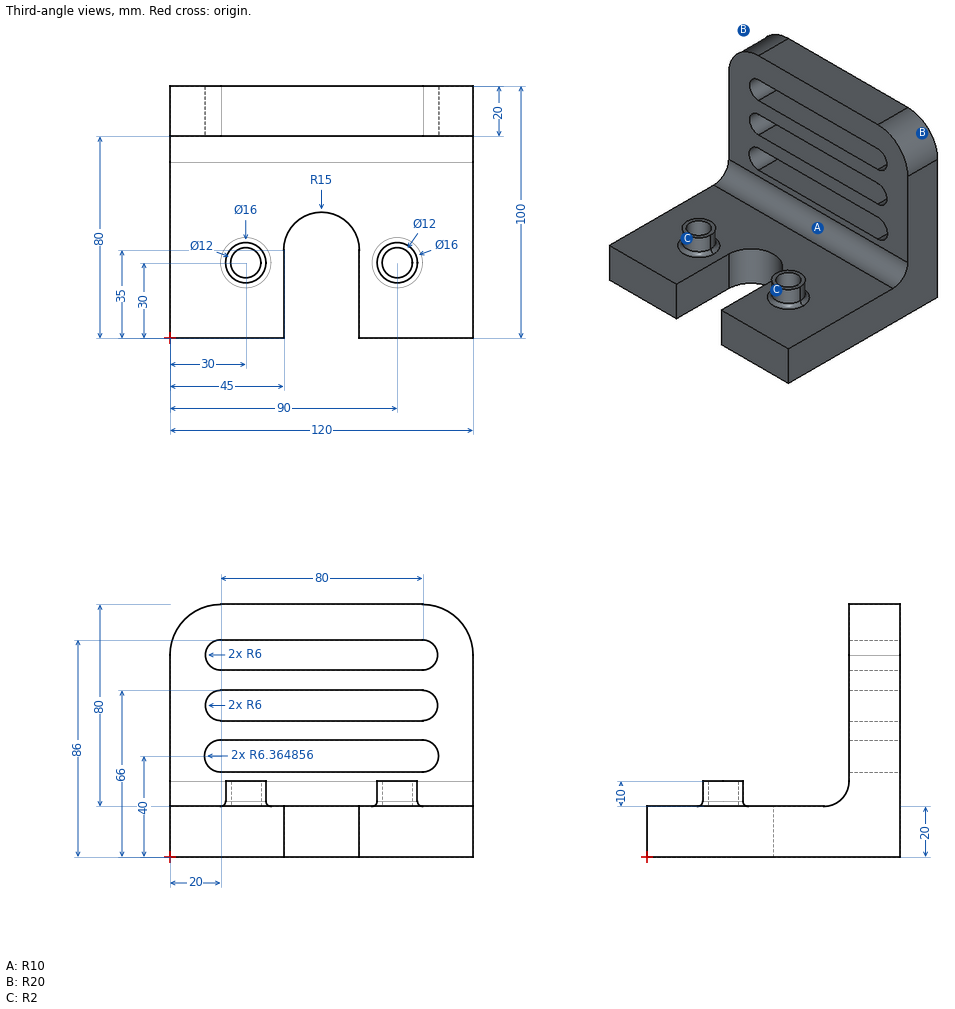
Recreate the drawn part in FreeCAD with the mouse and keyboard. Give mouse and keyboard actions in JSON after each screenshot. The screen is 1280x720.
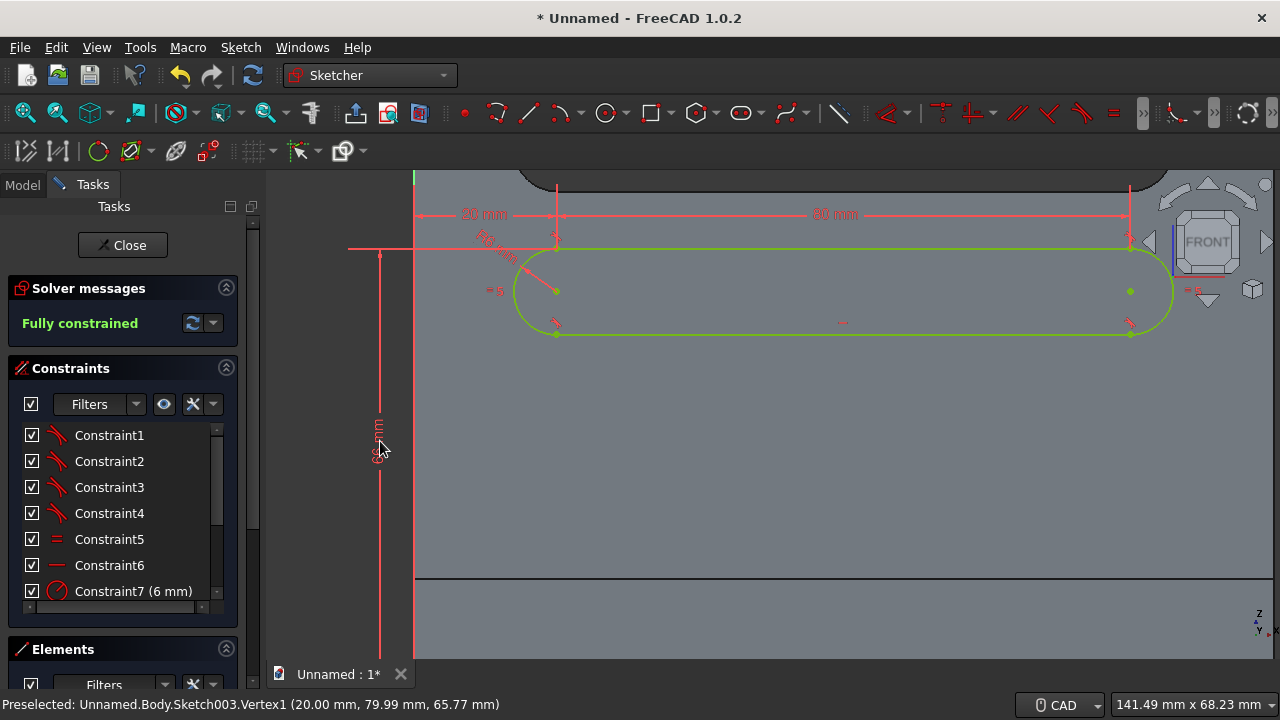
{"action": "left_click", "coordinate": [123, 245]}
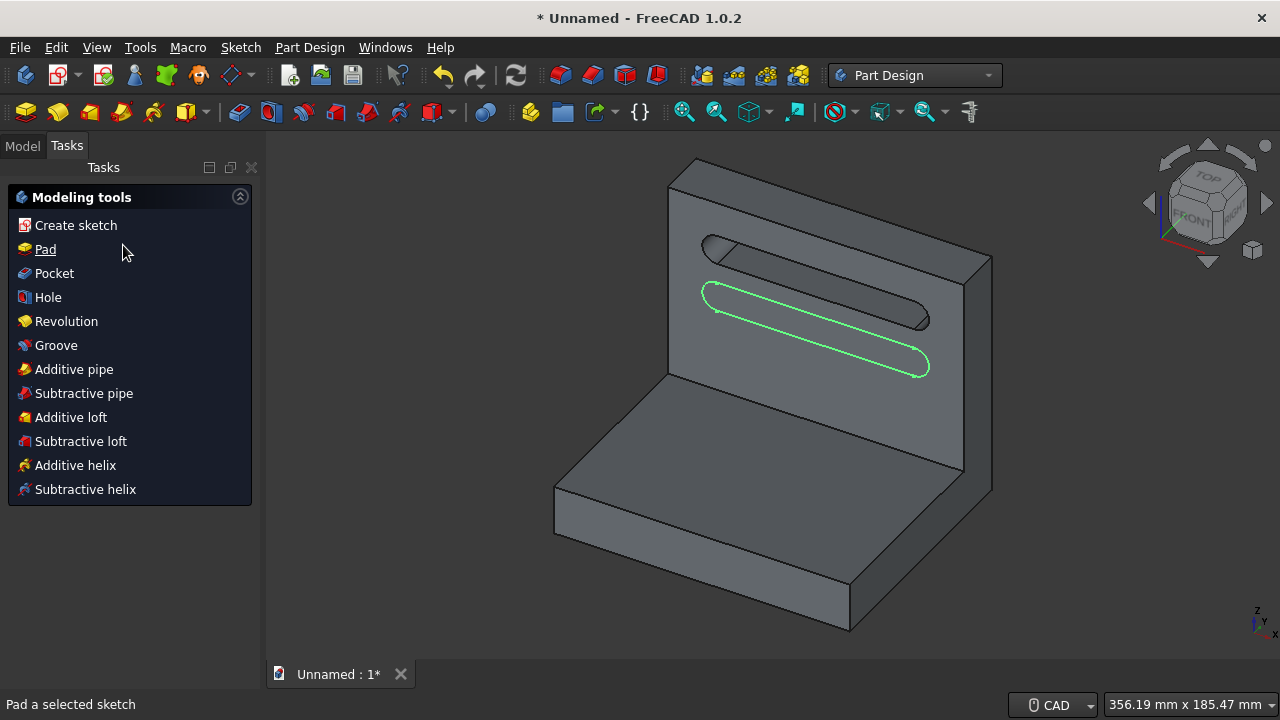
{"action": "left_click", "coordinate": [240, 112]}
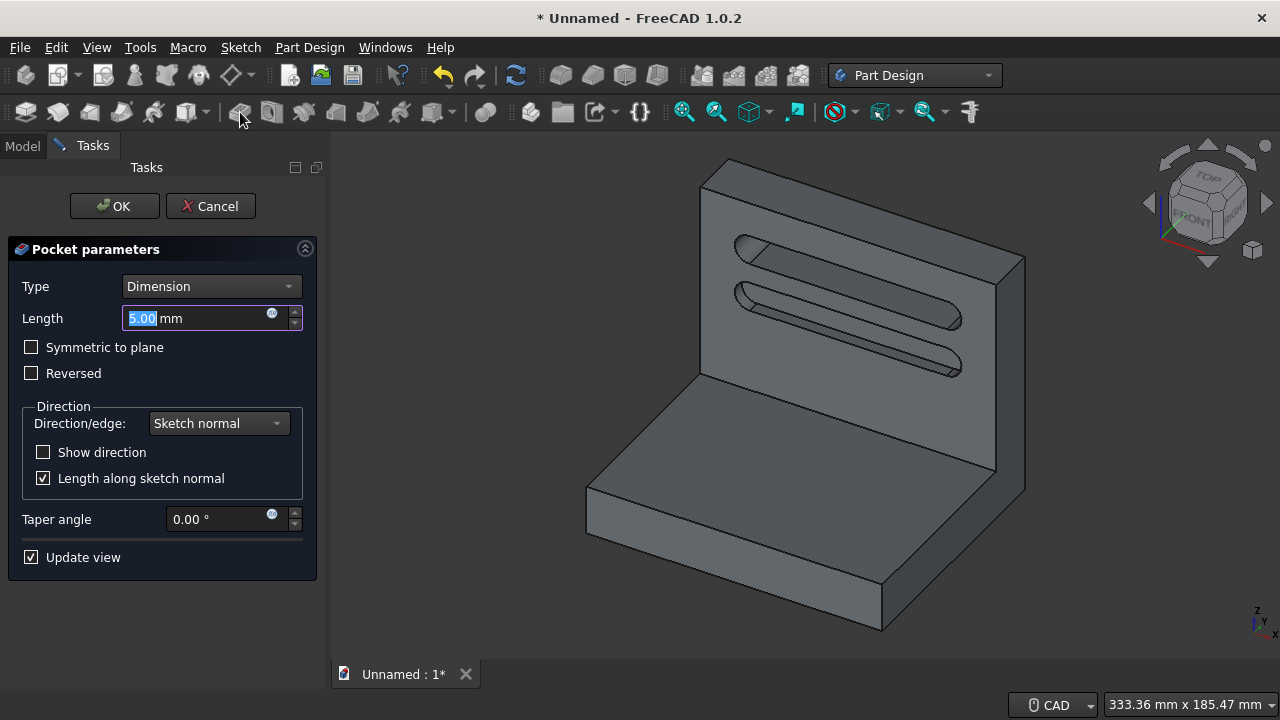
{"action": "left_click", "coordinate": [212, 286]}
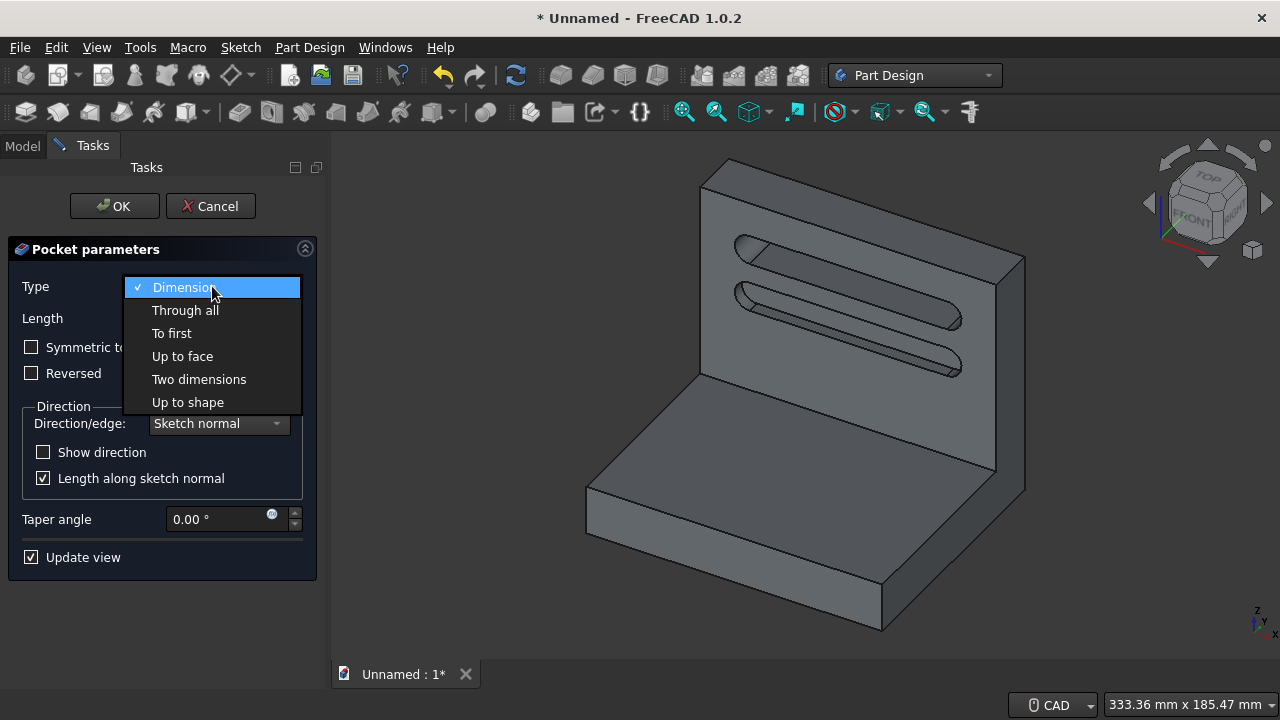
{"action": "left_click", "coordinate": [212, 310]}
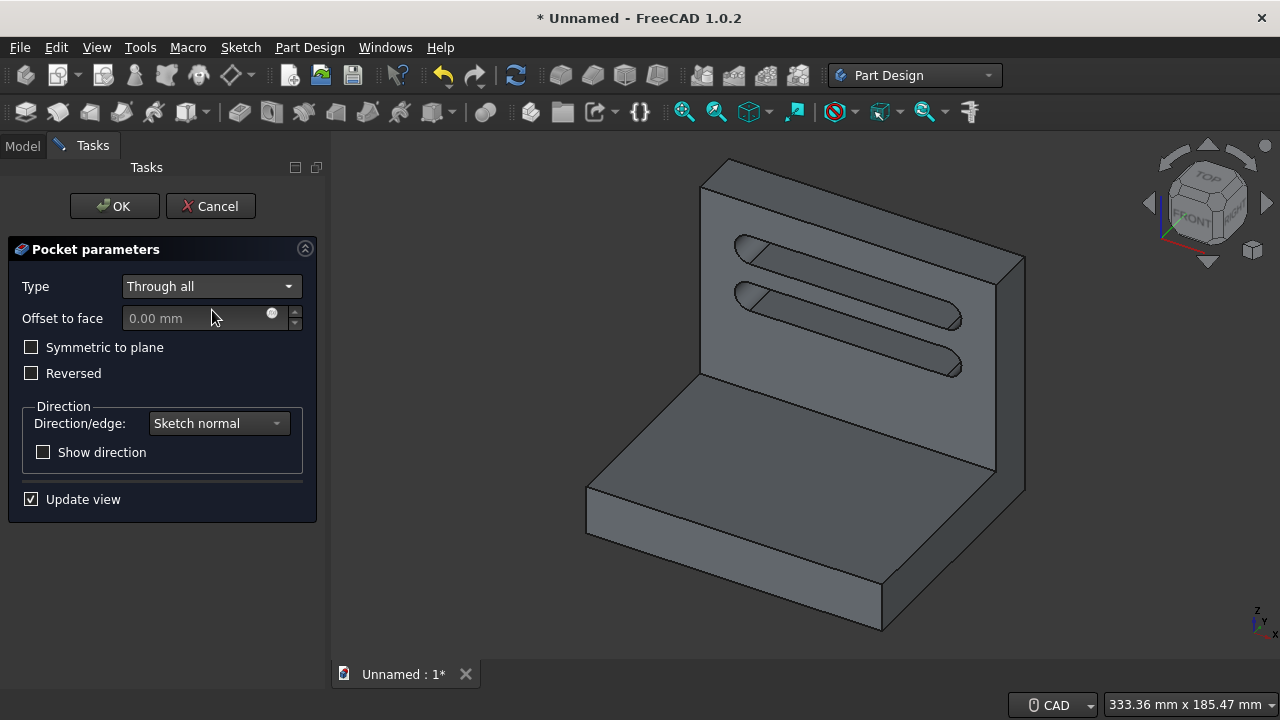
{"action": "left_click", "coordinate": [115, 206]}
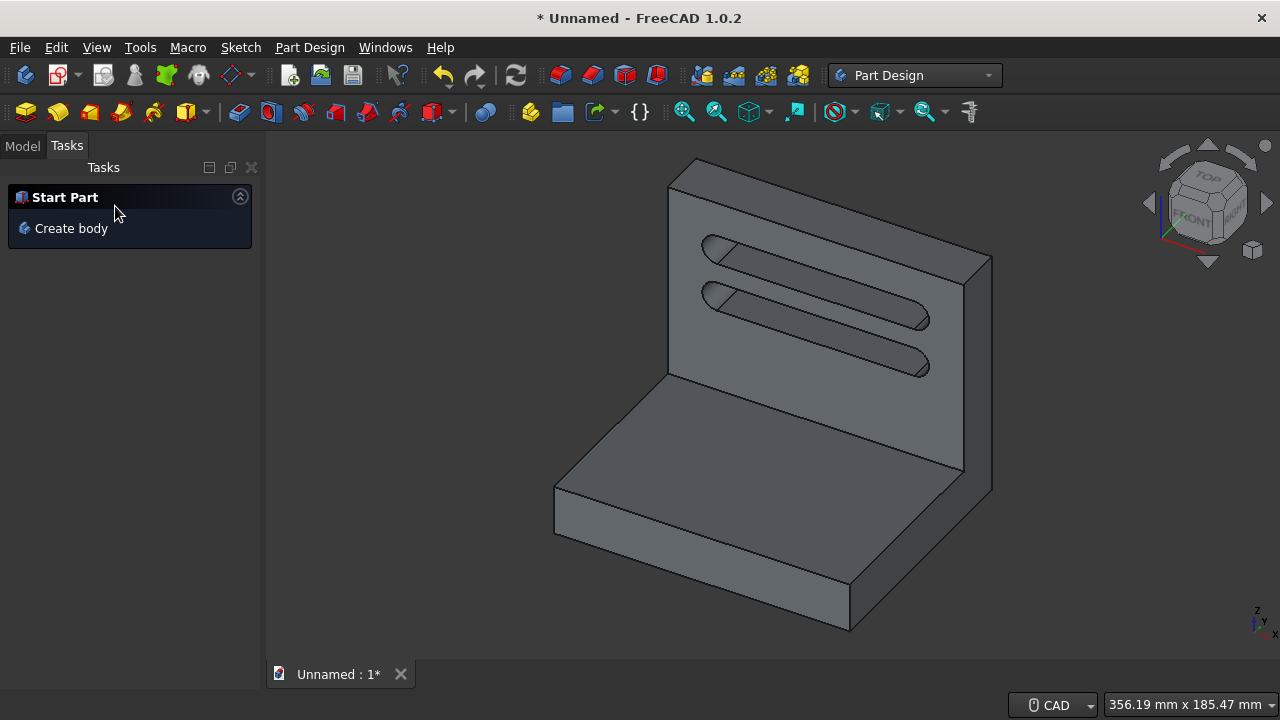
{"action": "left_click", "coordinate": [900, 410]}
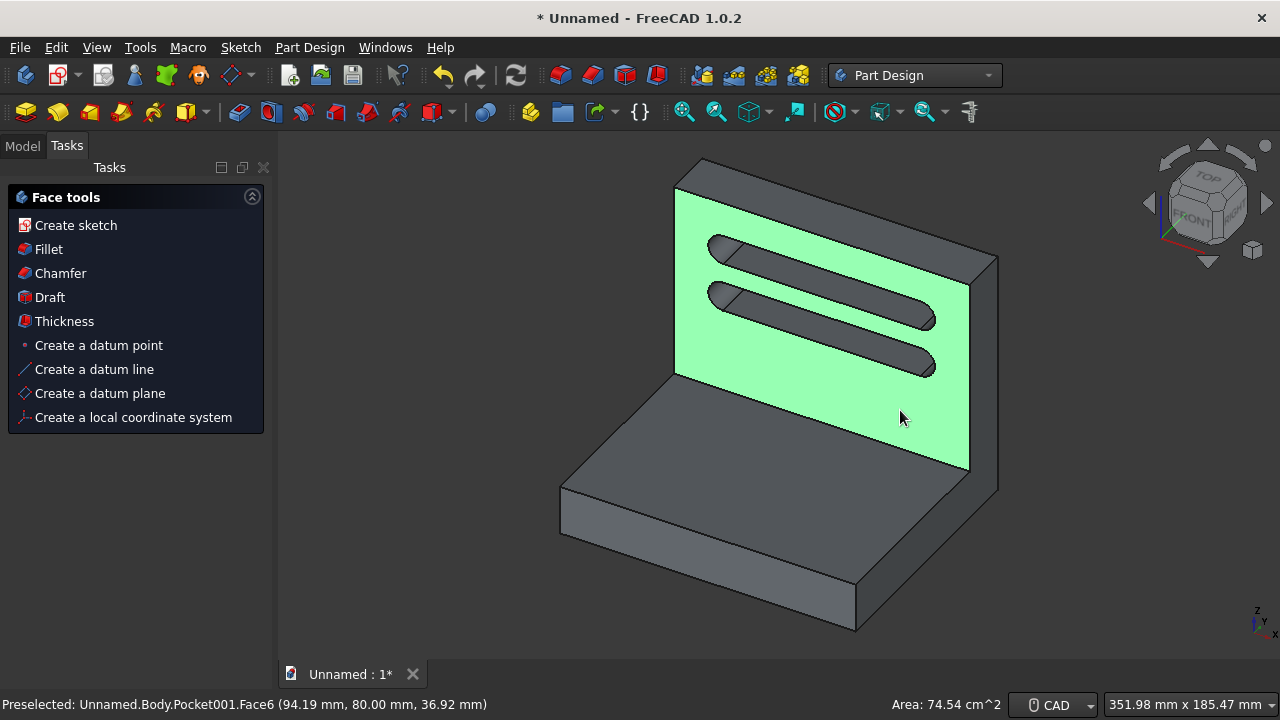
{"action": "left_click", "coordinate": [58, 76]}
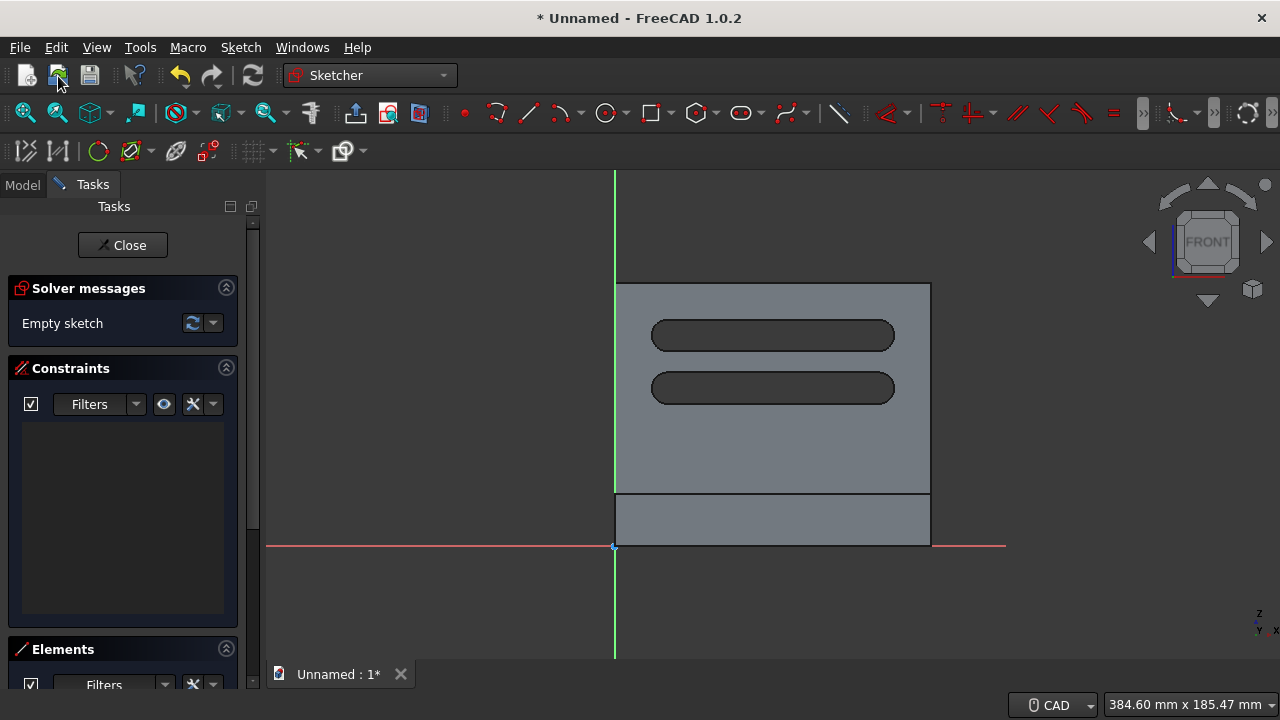
{"action": "scroll", "coordinate": [796, 543], "scroll_direction": "up", "scroll_amount": 4}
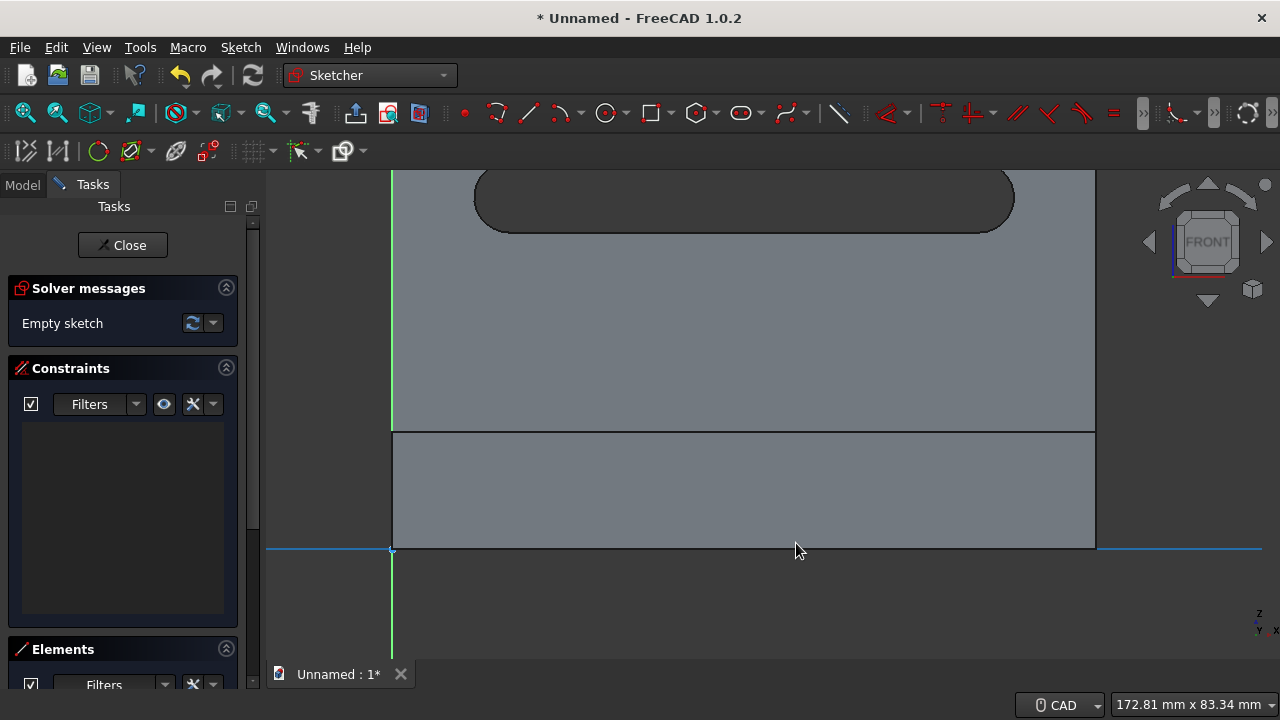
{"action": "left_click", "coordinate": [742, 114]}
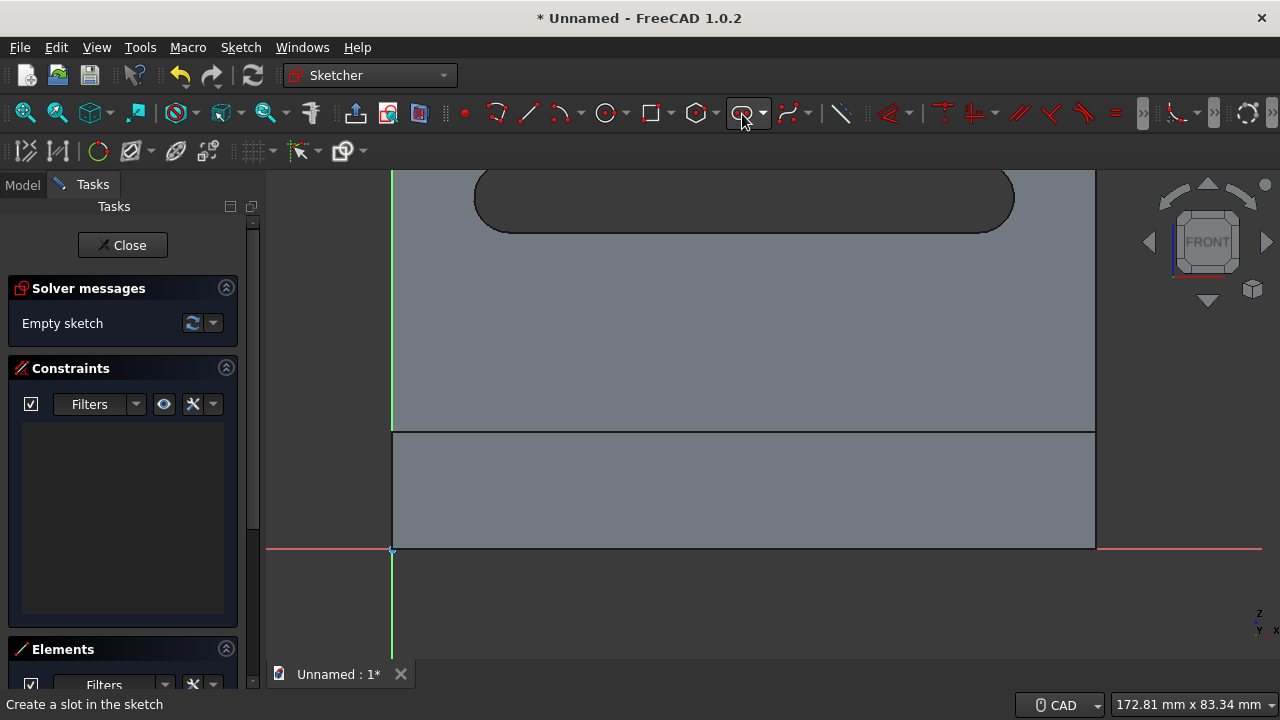
{"action": "left_click", "coordinate": [509, 315]}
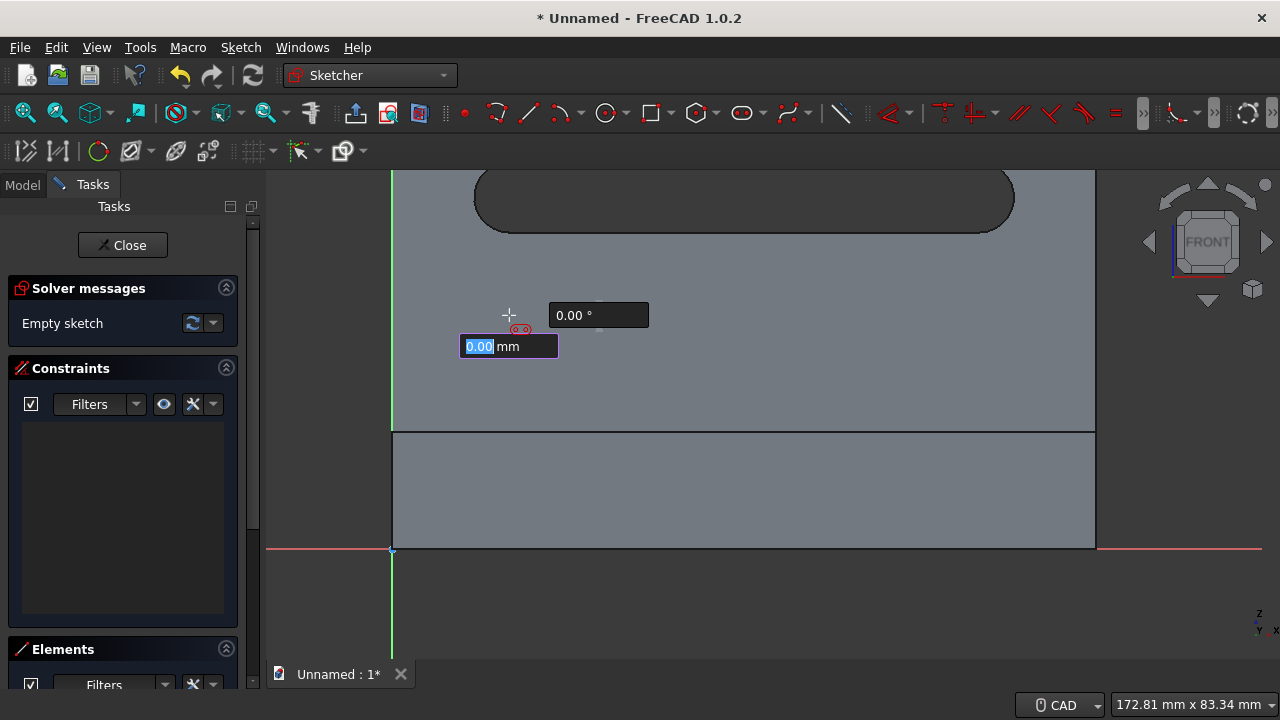
{"action": "left_click", "coordinate": [979, 315]}